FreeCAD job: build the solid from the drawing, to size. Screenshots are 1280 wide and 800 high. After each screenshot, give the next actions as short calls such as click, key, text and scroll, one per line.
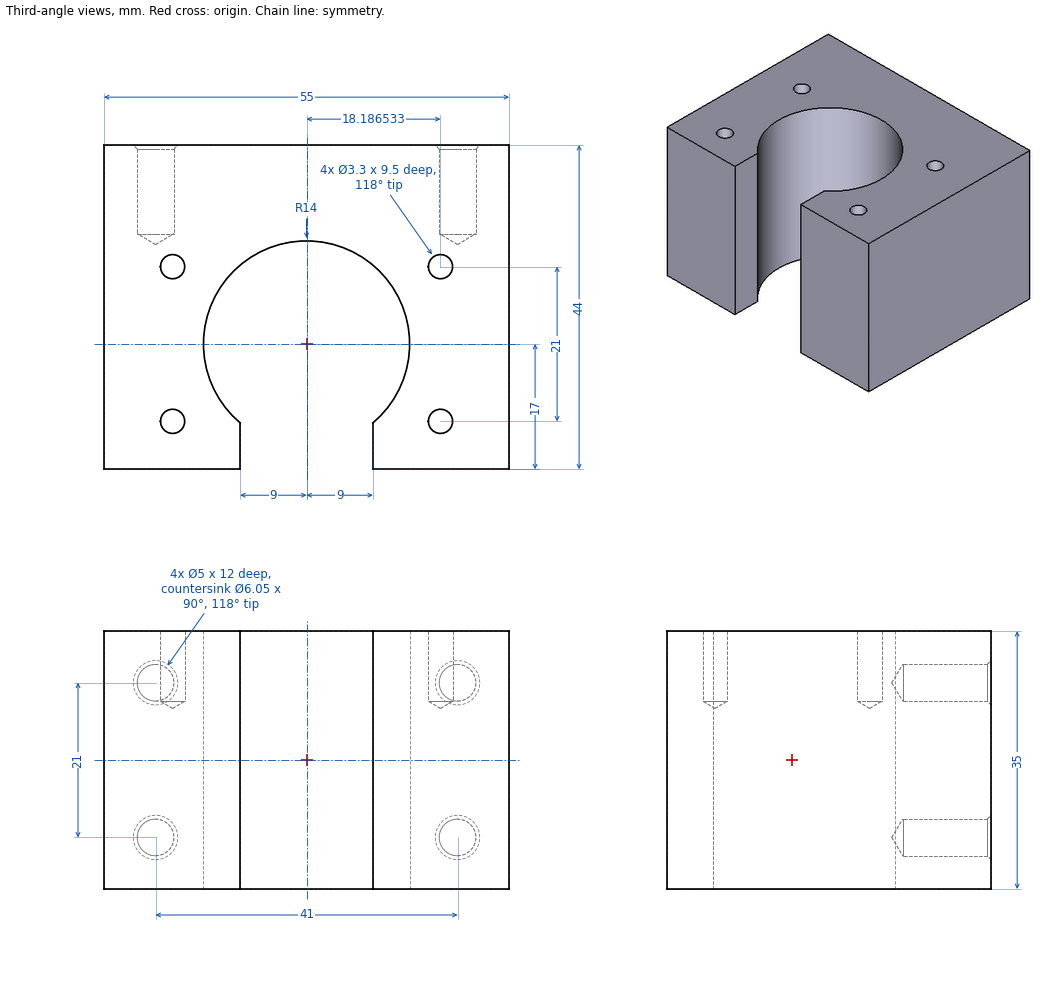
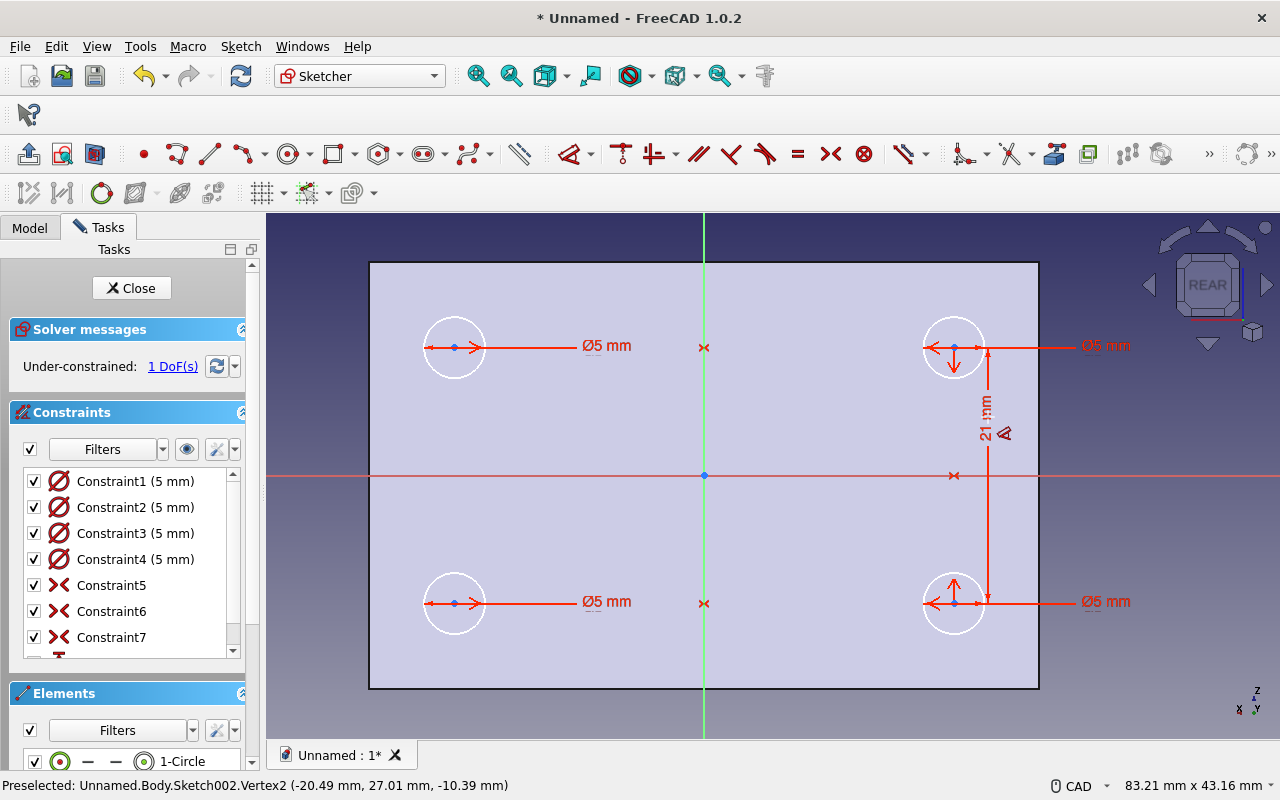
click(954, 604)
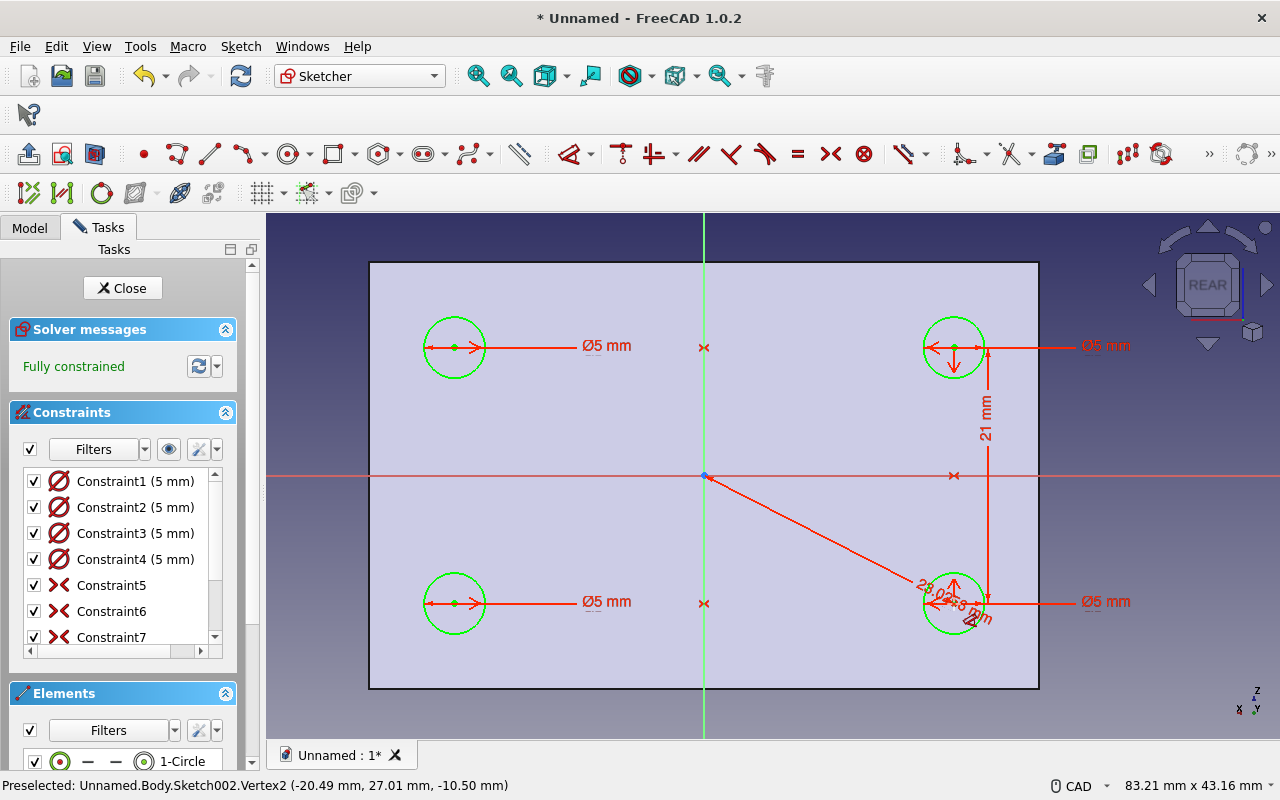
click(455, 604)
click(589, 638)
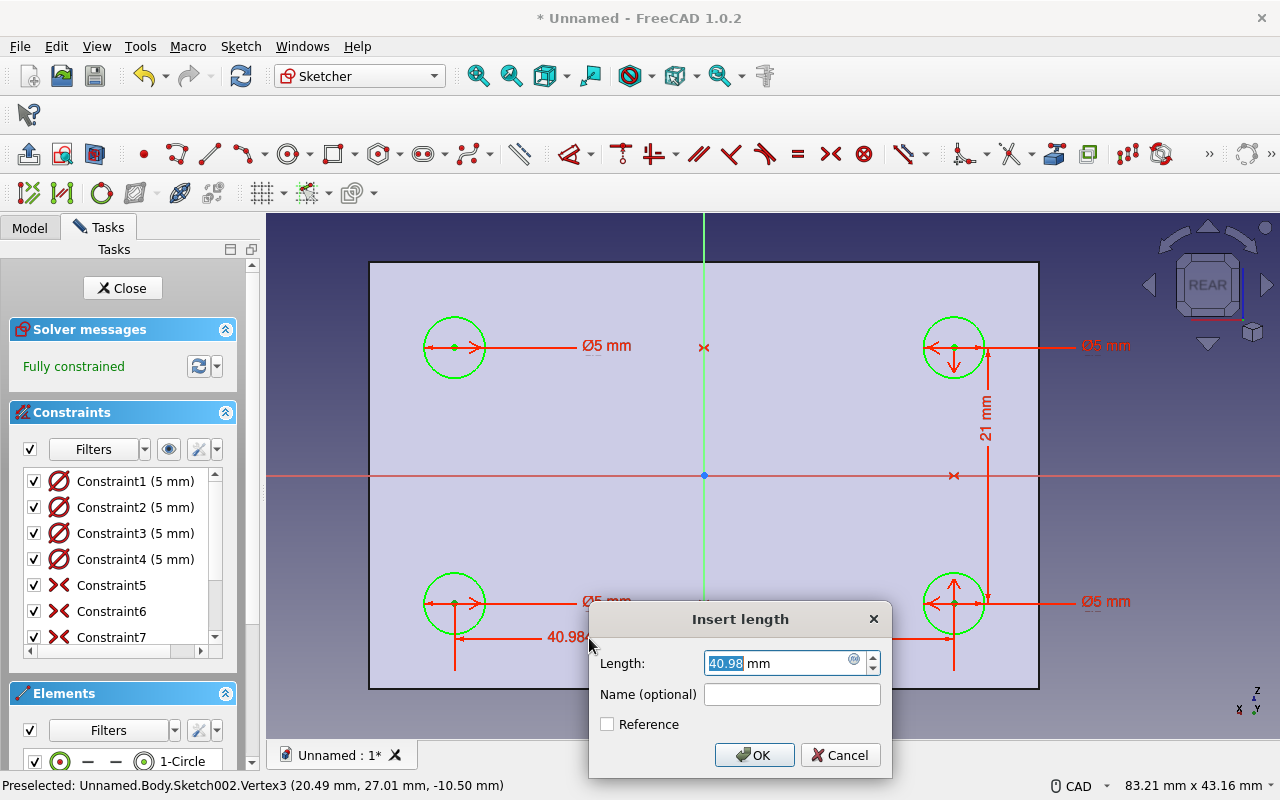
text(41)
key(Return)
key(Escape)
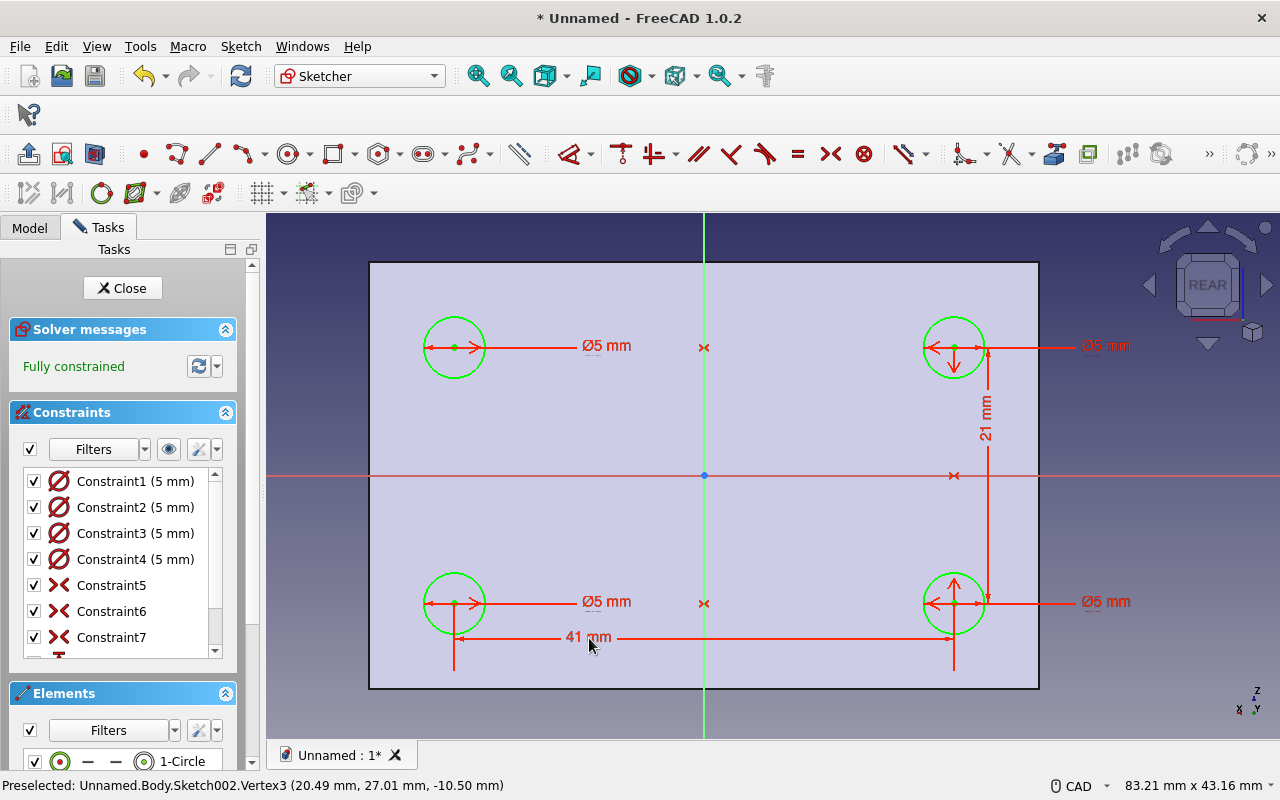
click(123, 288)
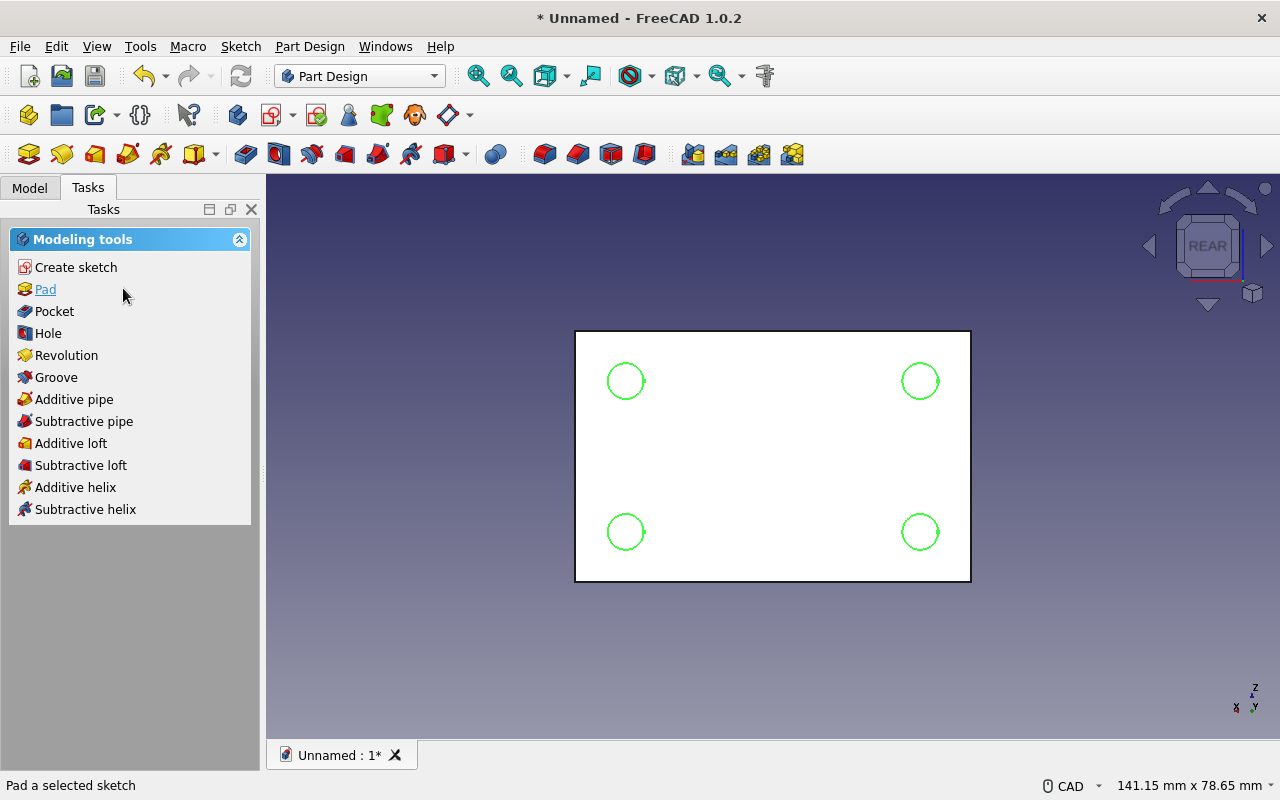
click(279, 154)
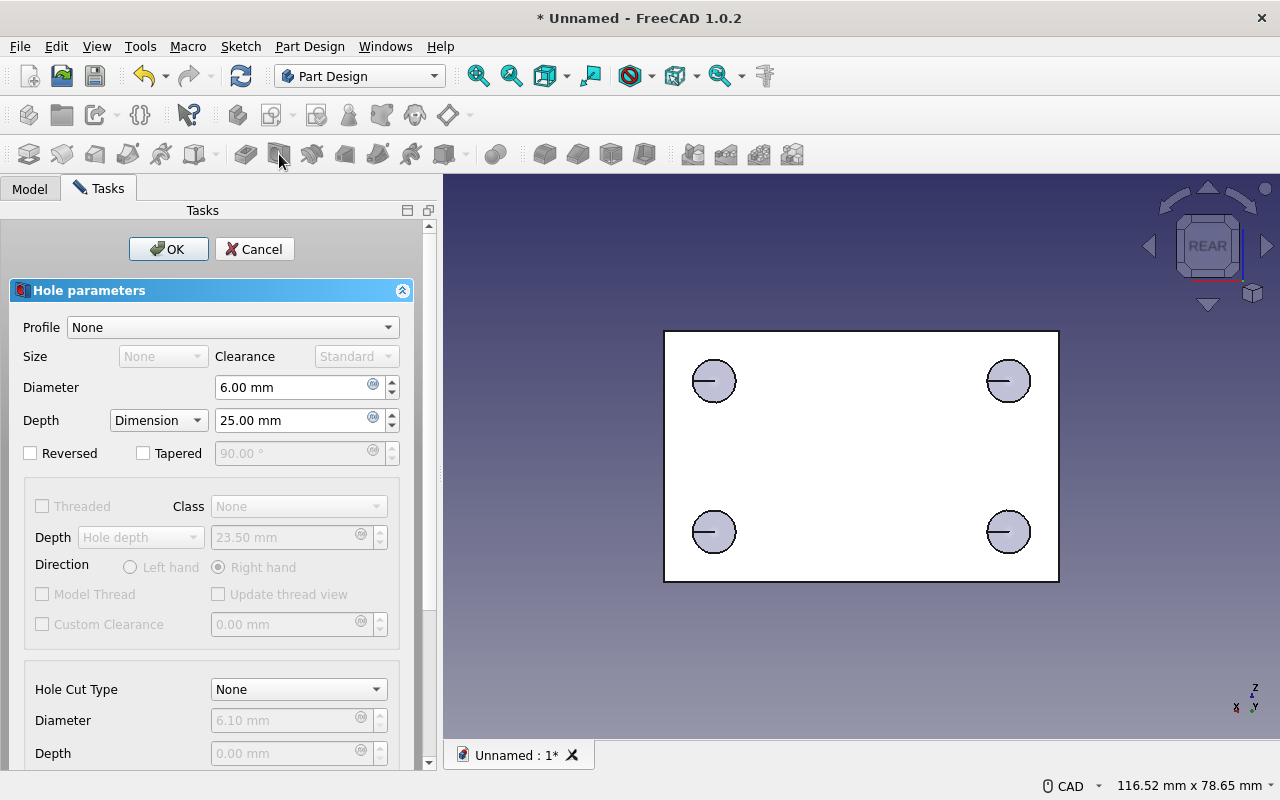
triple_click(300, 388)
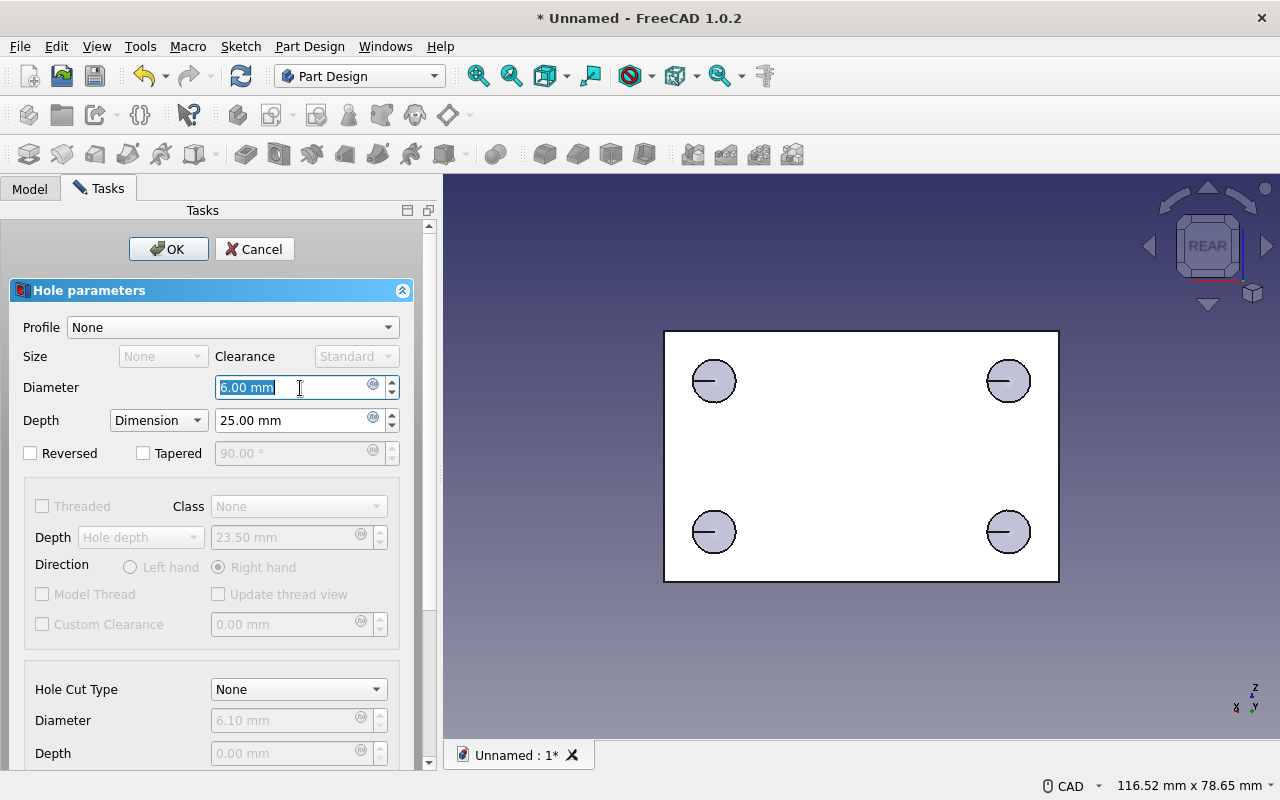
text(5)
key(Tab)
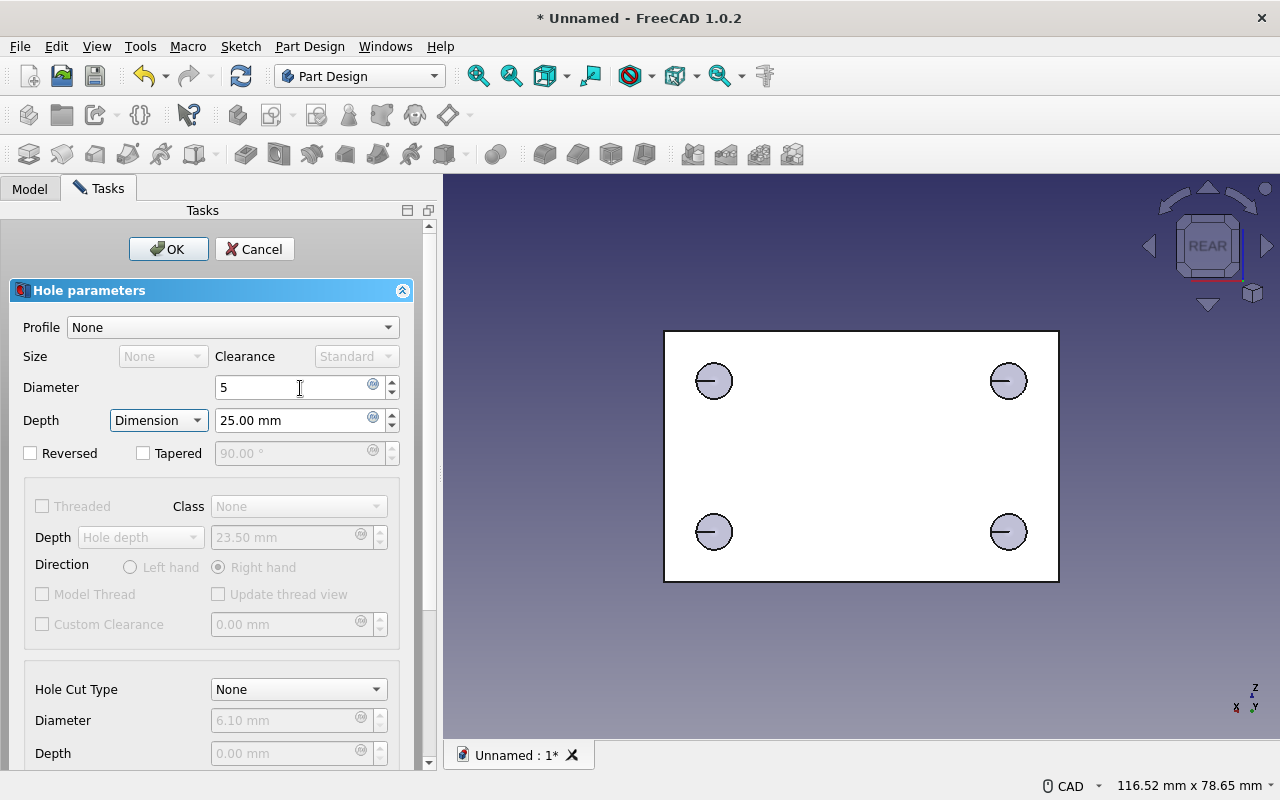
triple_click(300, 420)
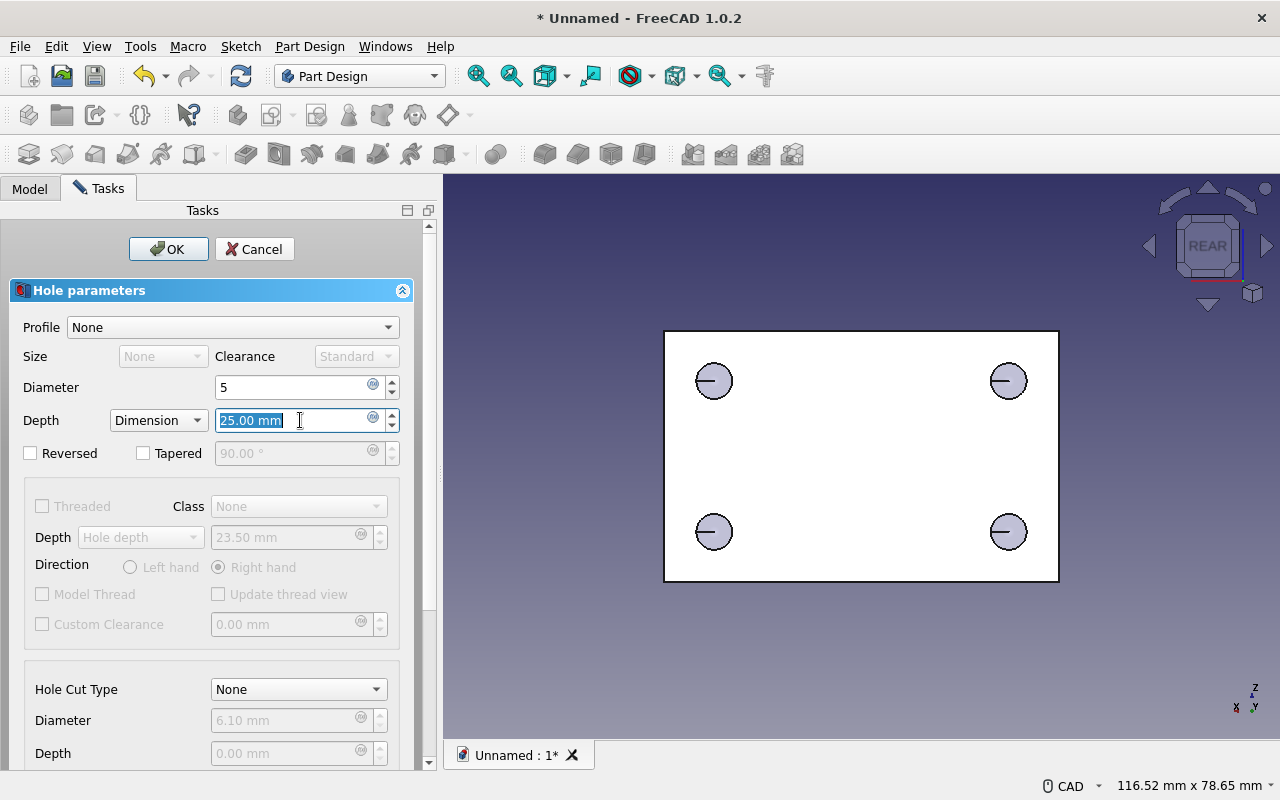
text(12)
key(Tab)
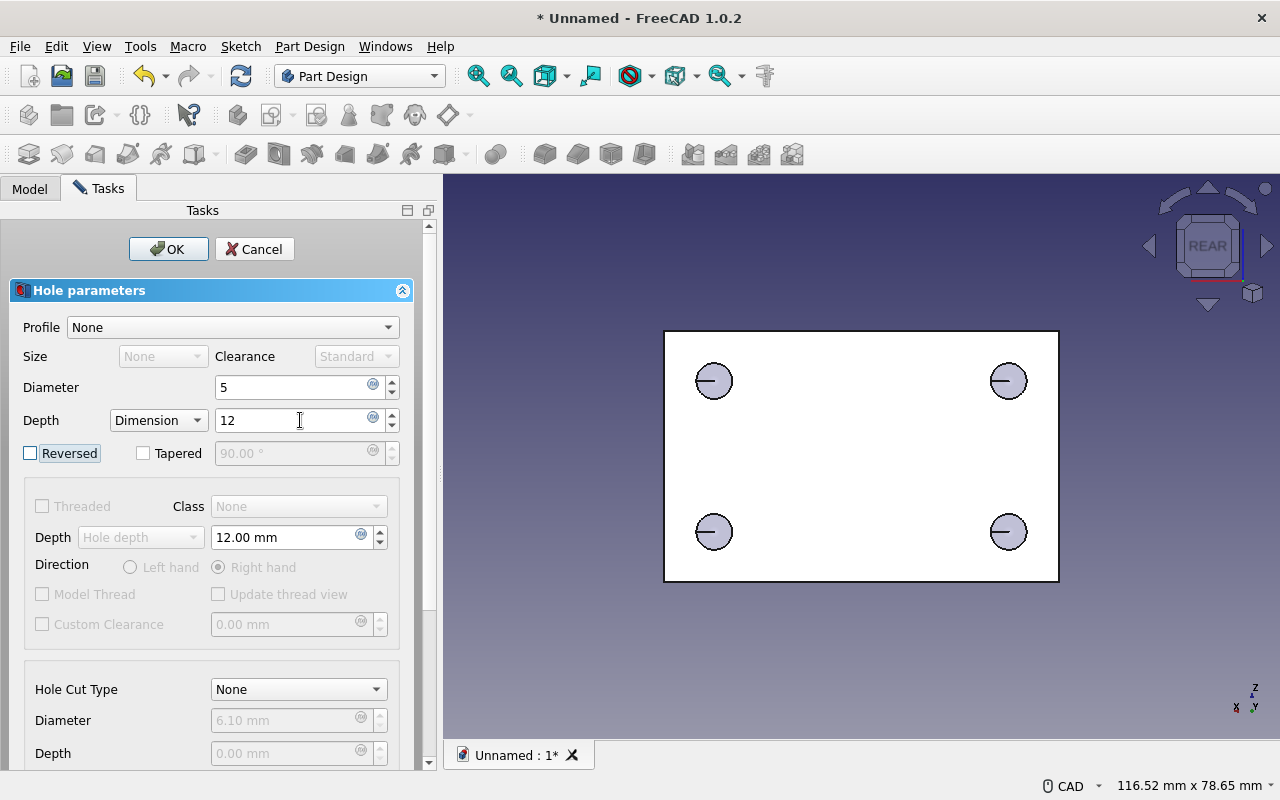
click(300, 690)